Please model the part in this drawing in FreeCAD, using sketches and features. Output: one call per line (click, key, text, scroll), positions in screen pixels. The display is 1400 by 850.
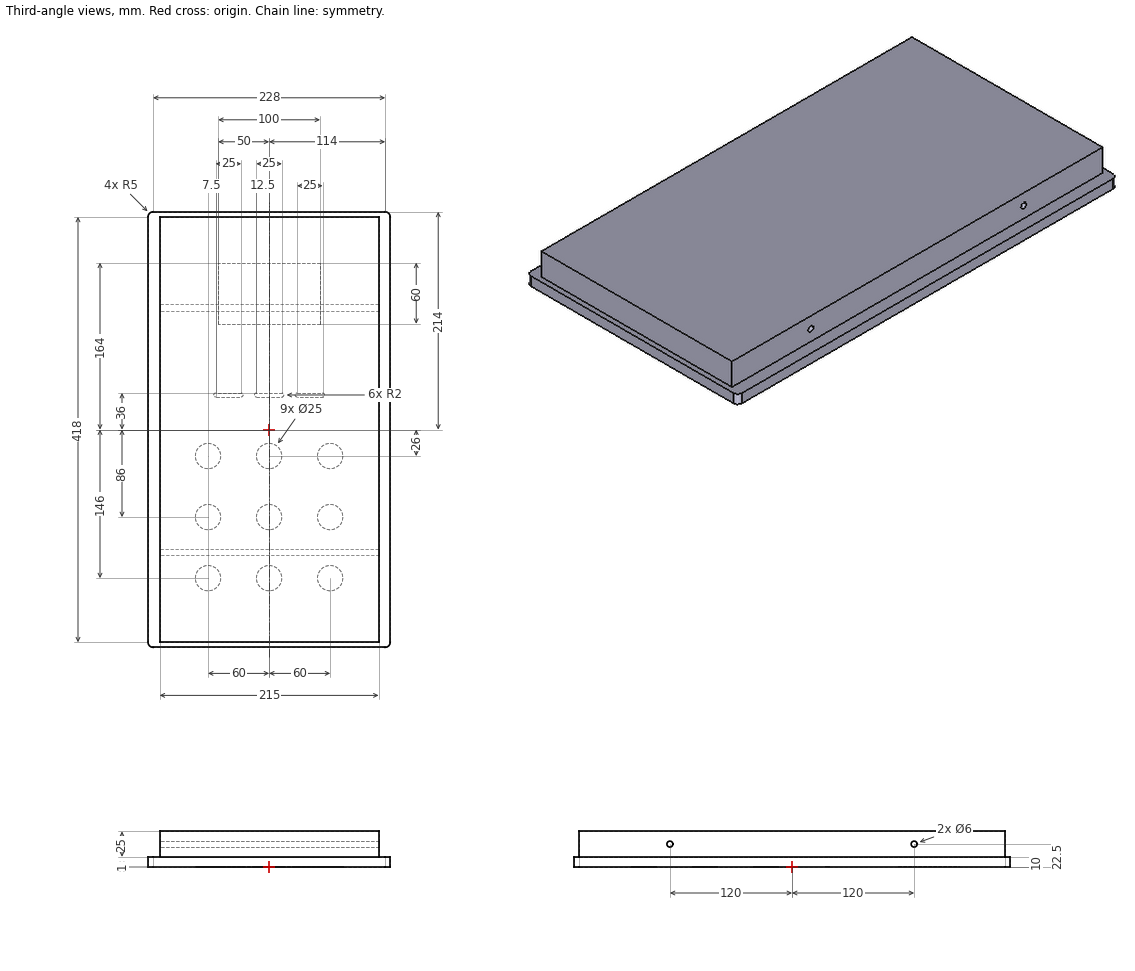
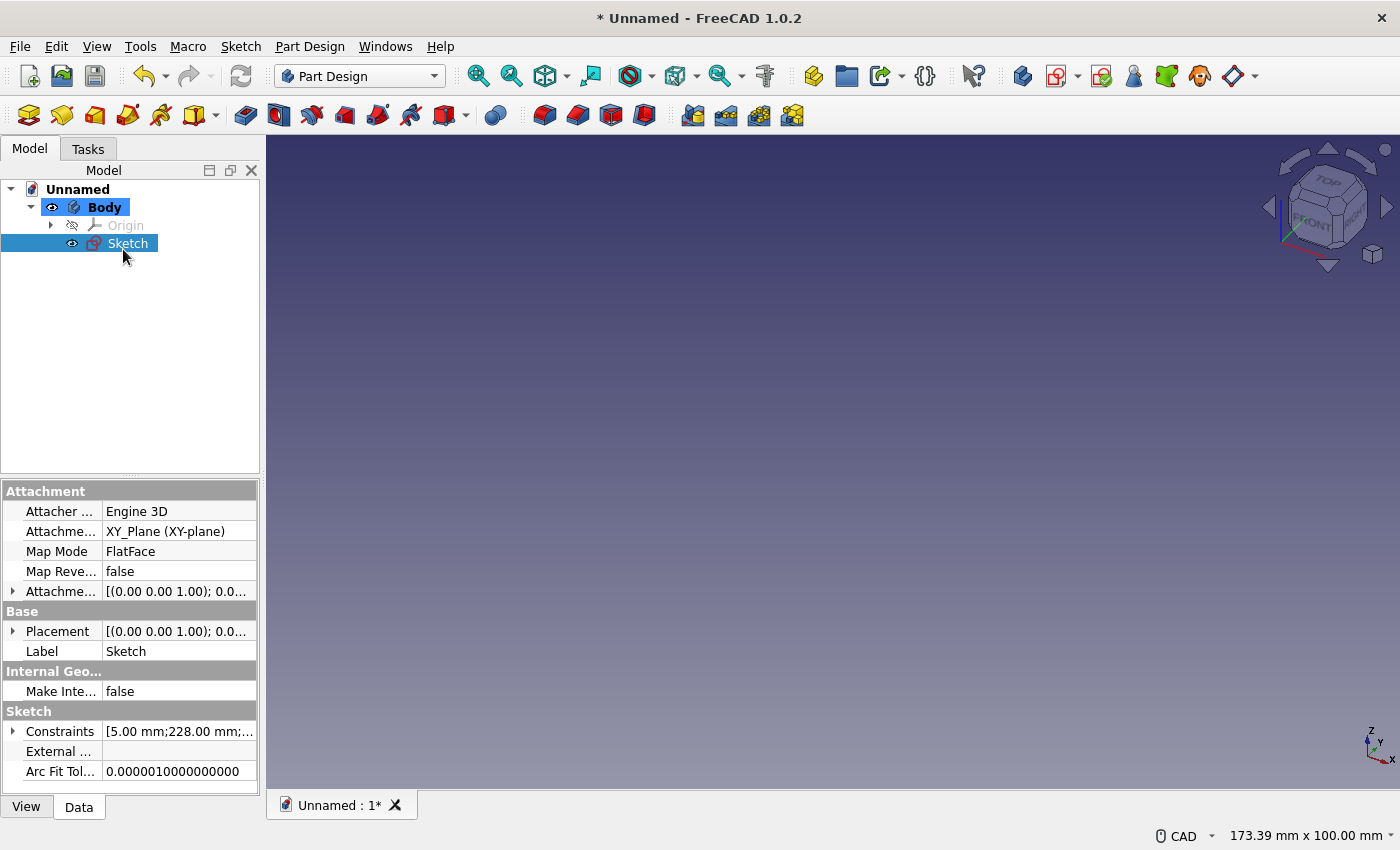
click(29, 116)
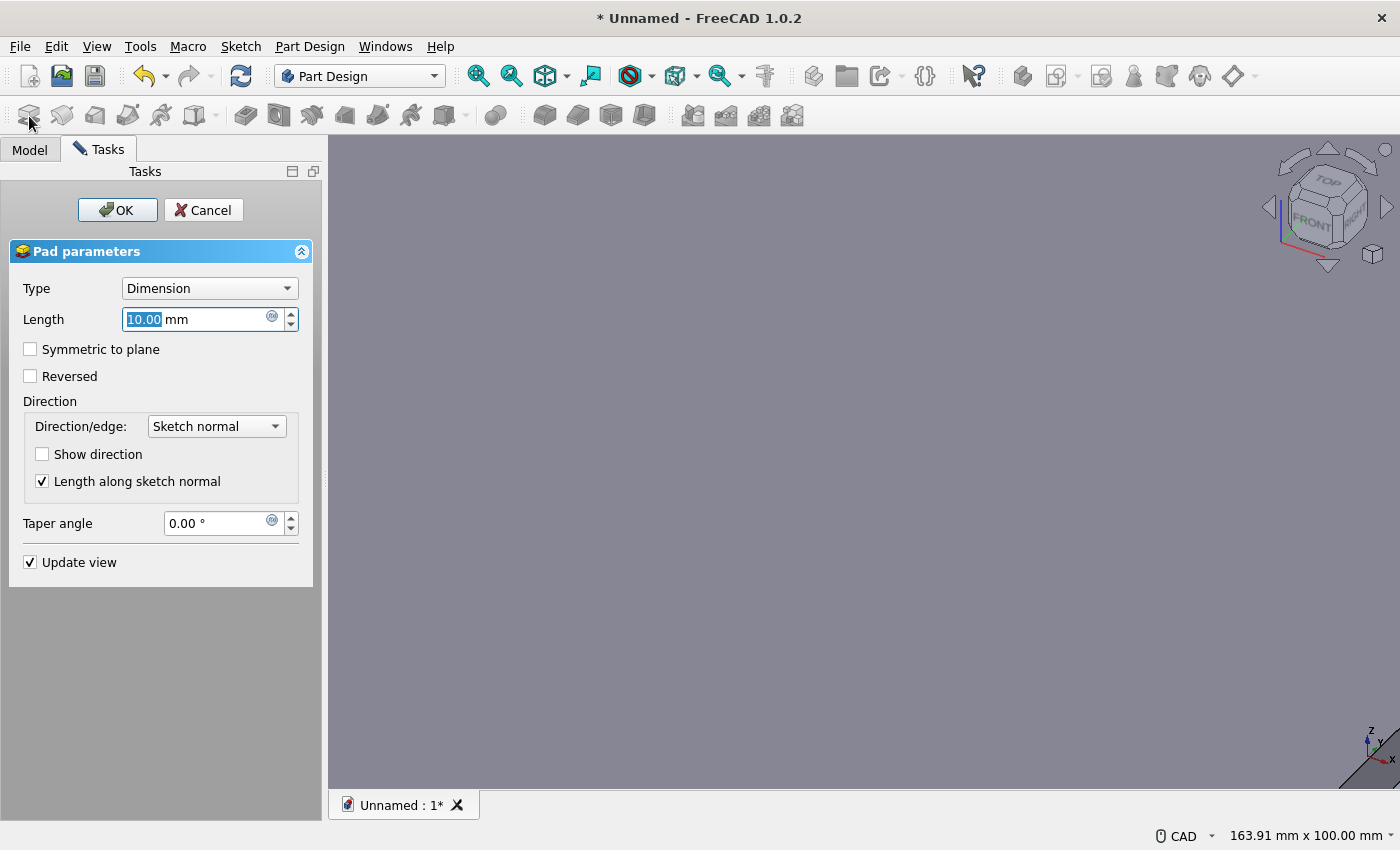
text(10)
key(Tab)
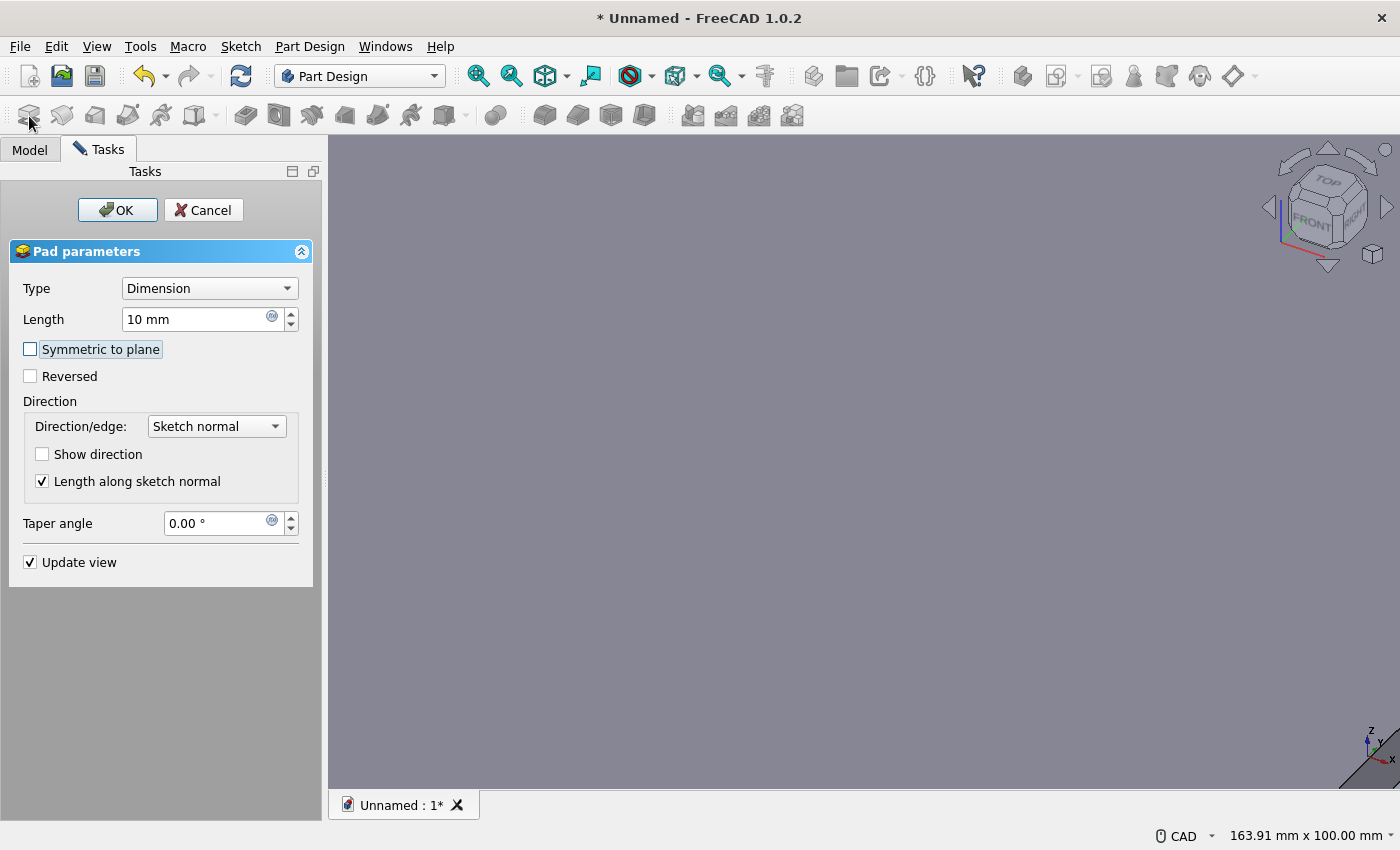
click(118, 210)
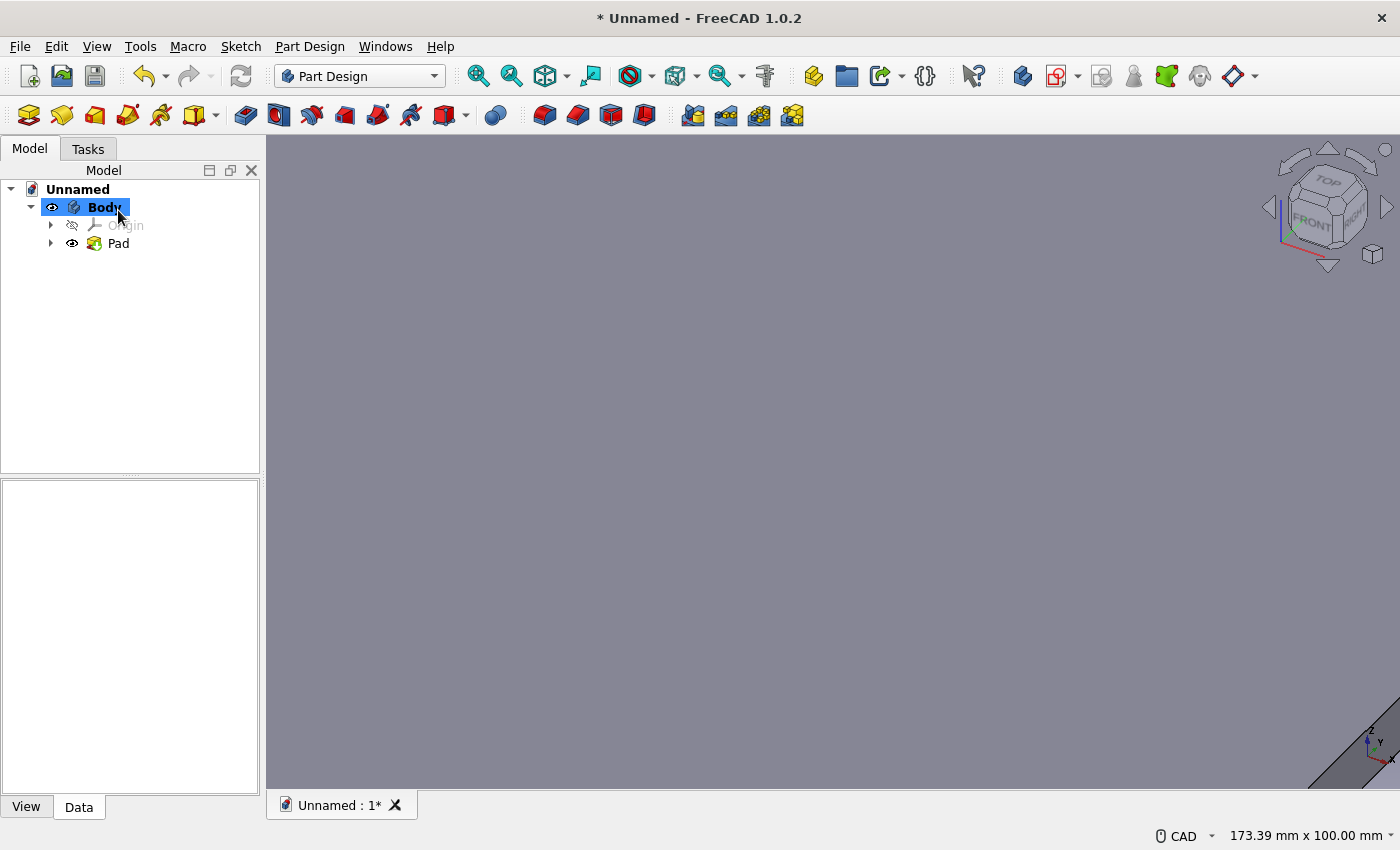
click(479, 76)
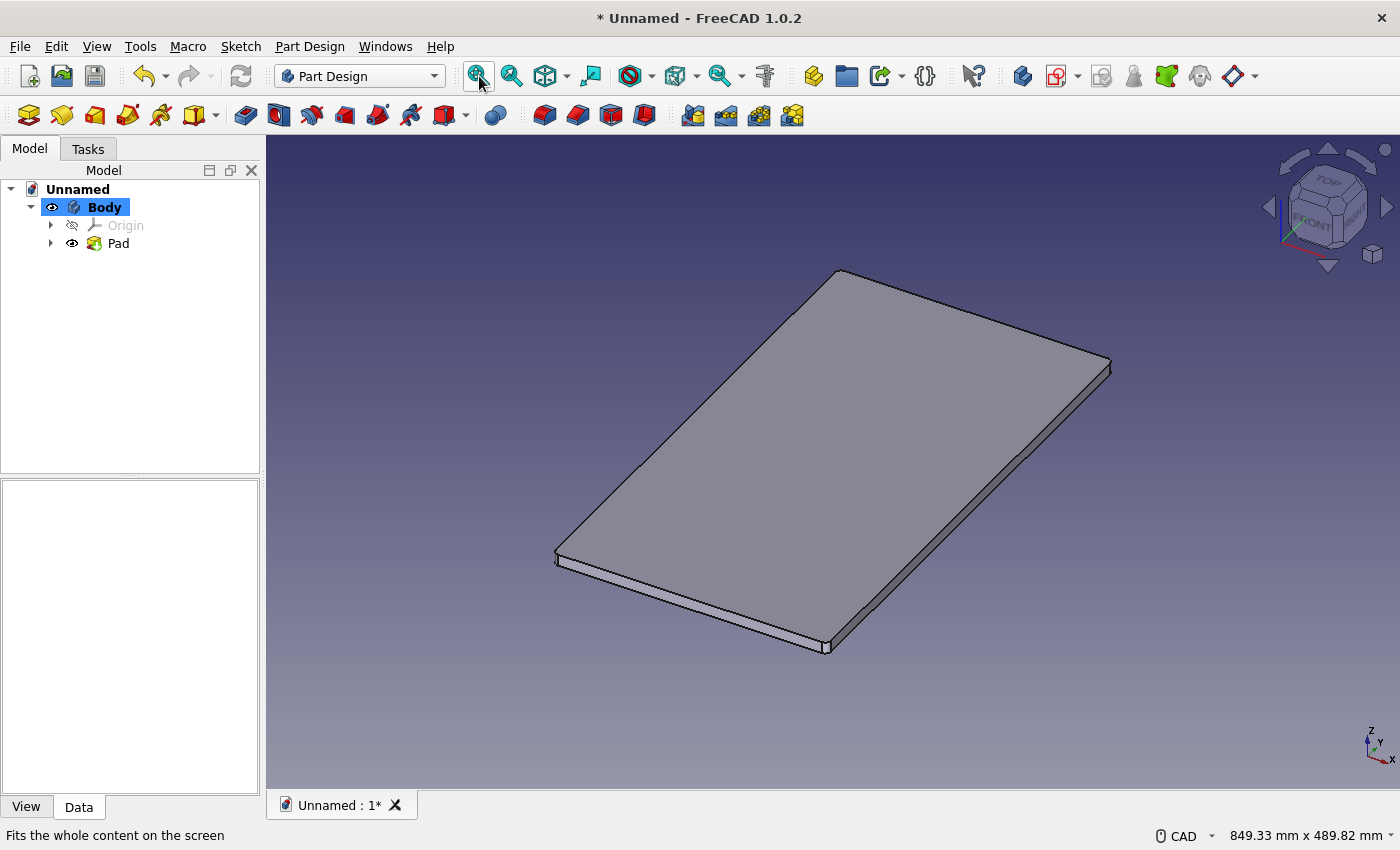
click(874, 415)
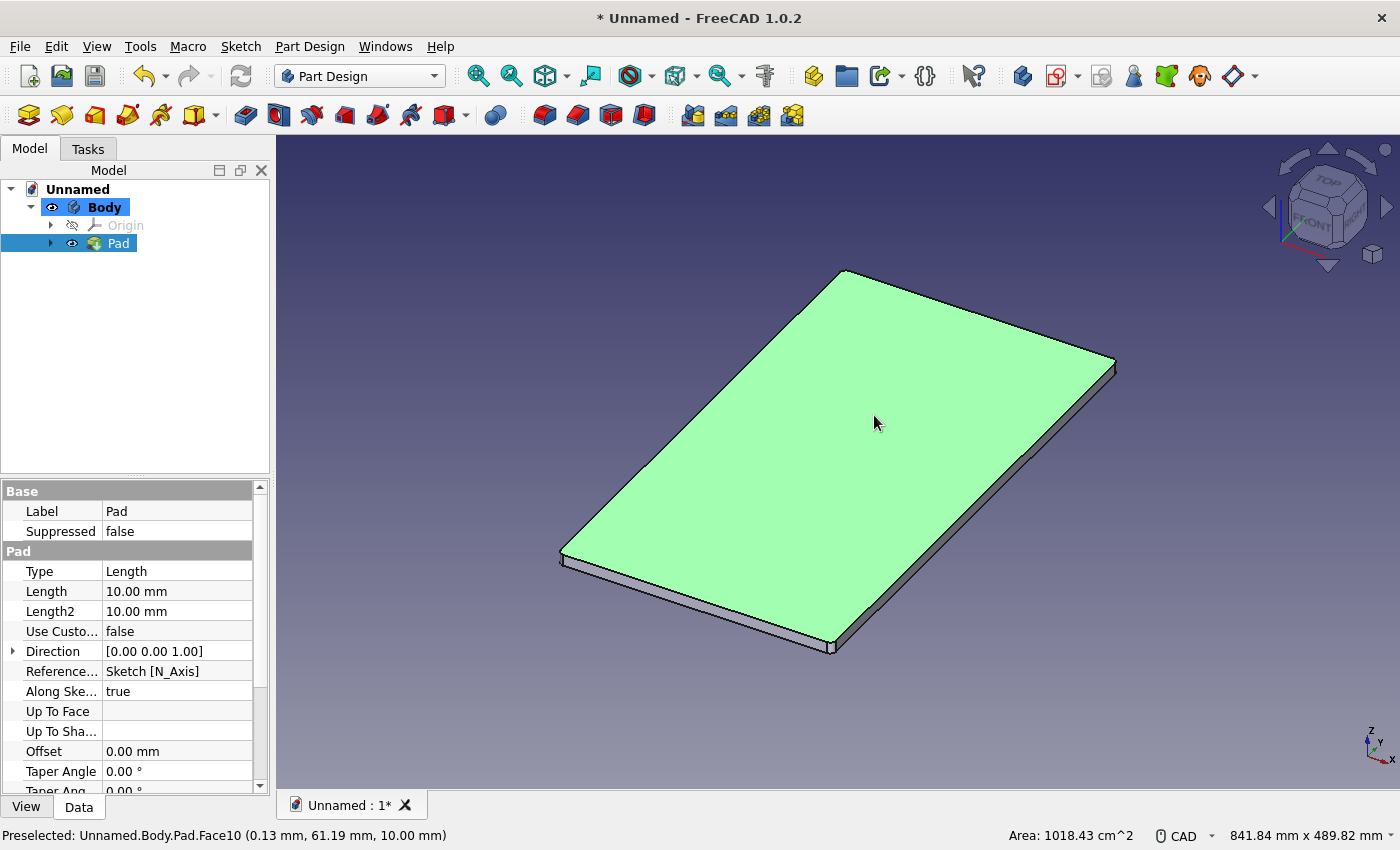
click(1056, 76)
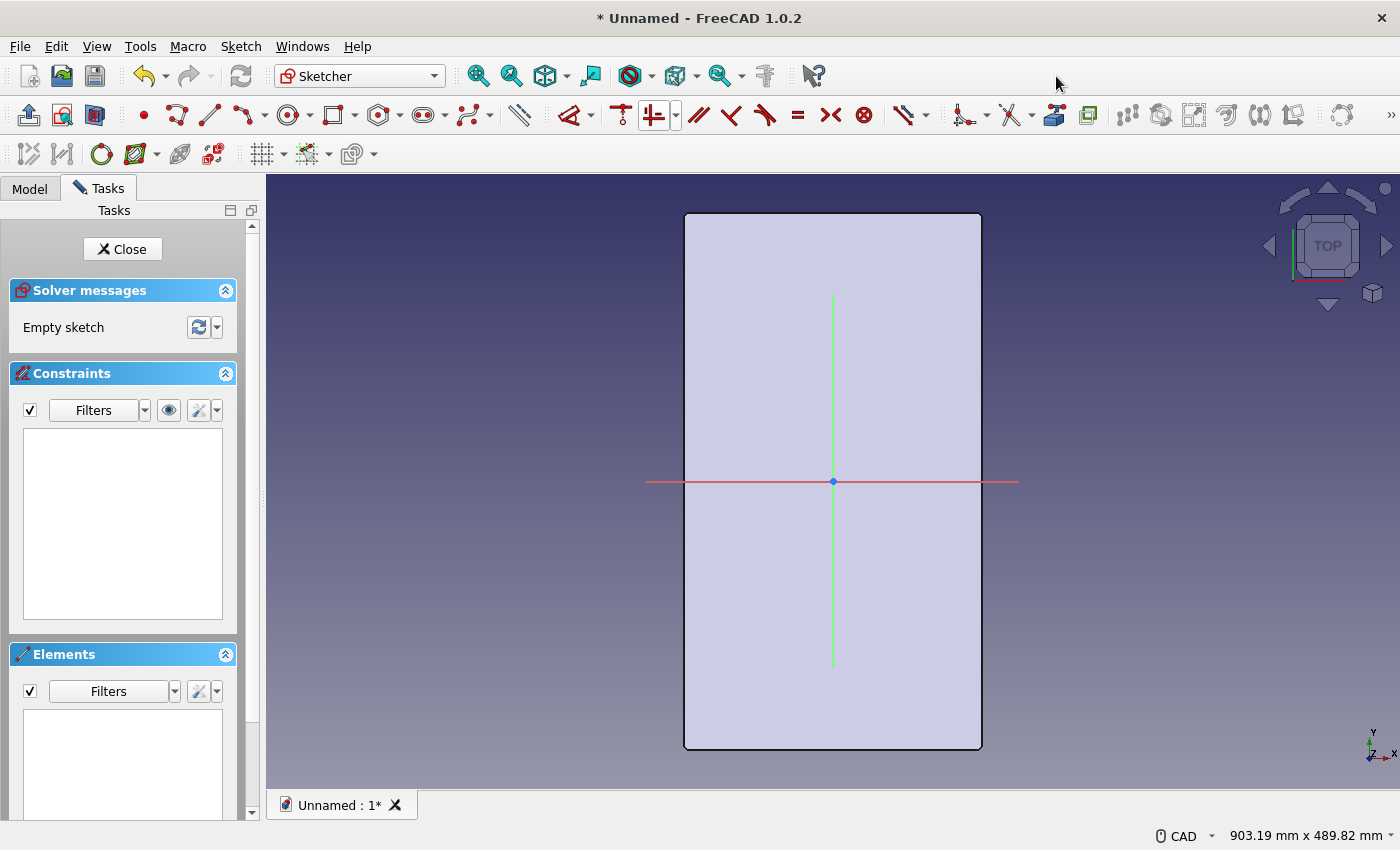
scroll(455, 482, down, 1)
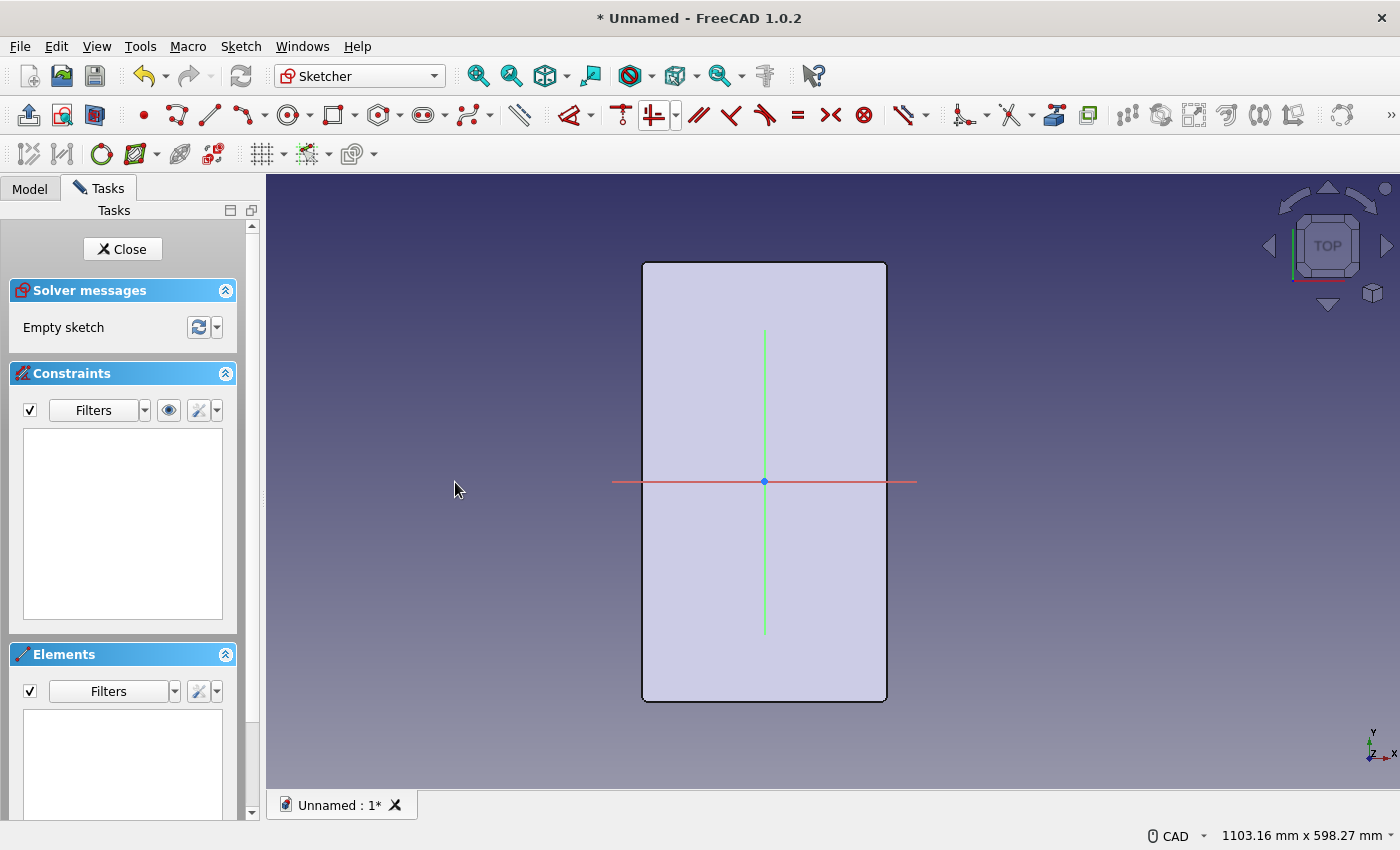
key(g)
key(v)